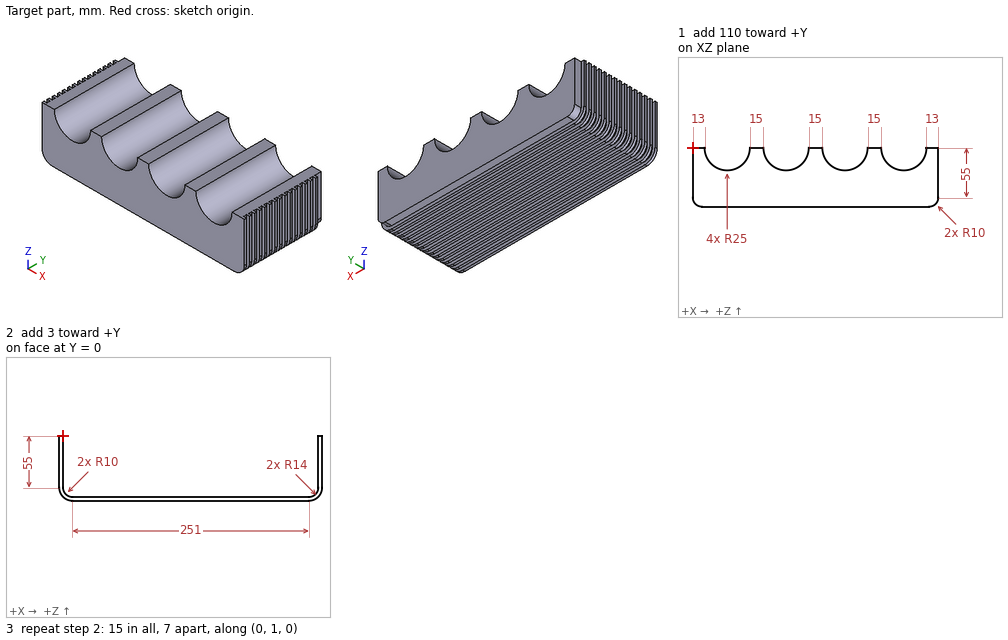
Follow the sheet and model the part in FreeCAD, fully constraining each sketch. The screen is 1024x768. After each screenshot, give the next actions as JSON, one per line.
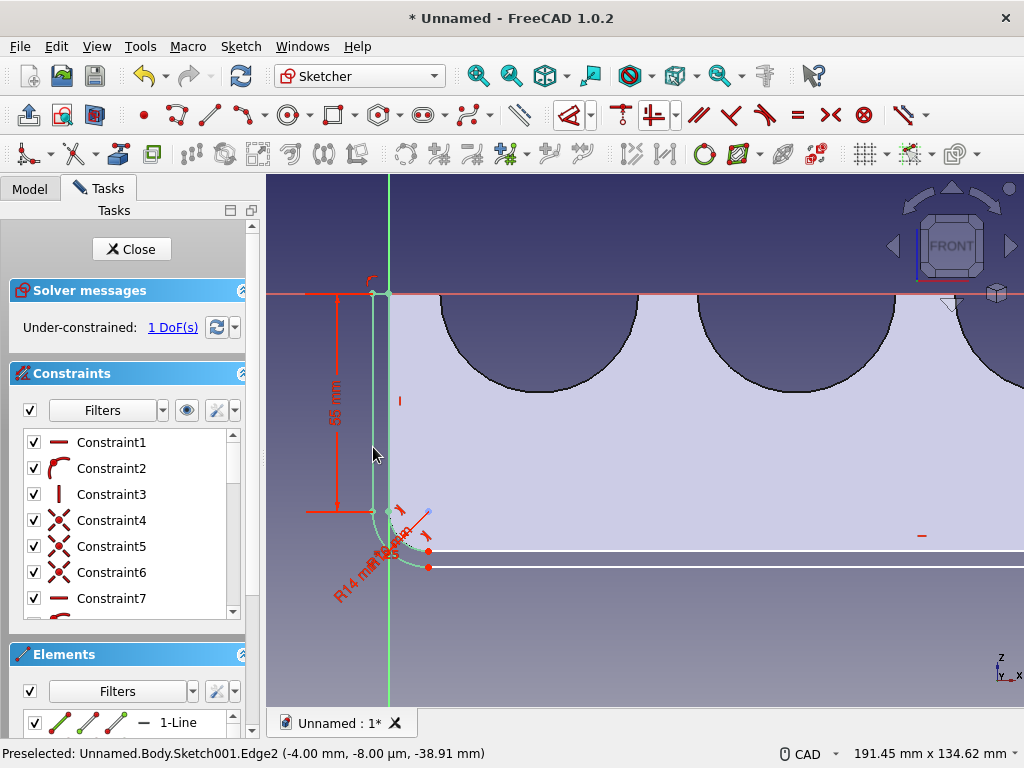
{"action": "left_click", "coordinate": [726, 567]}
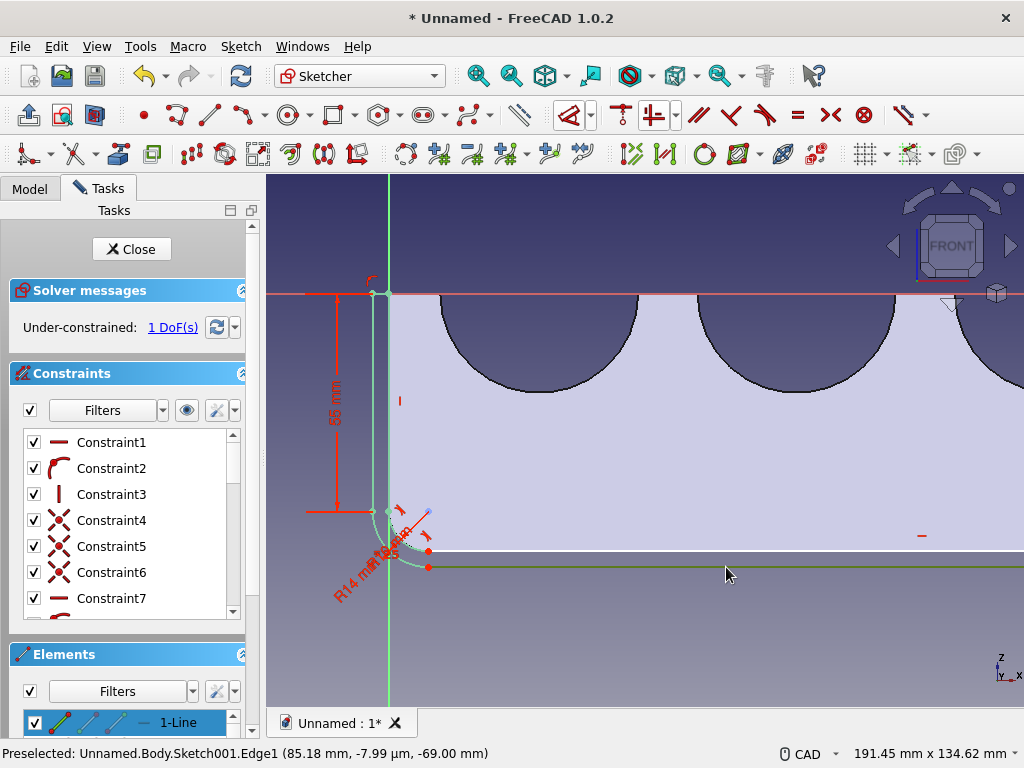
{"action": "key", "text": "l"}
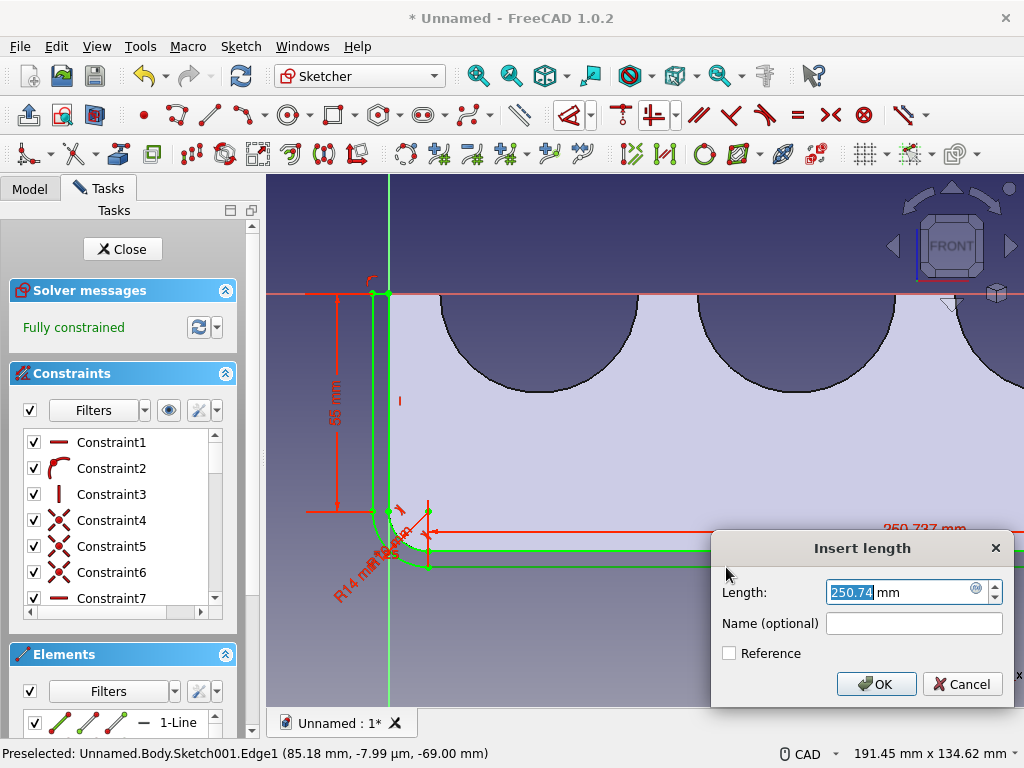
{"action": "type", "text": "251"}
{"action": "key", "text": "Return"}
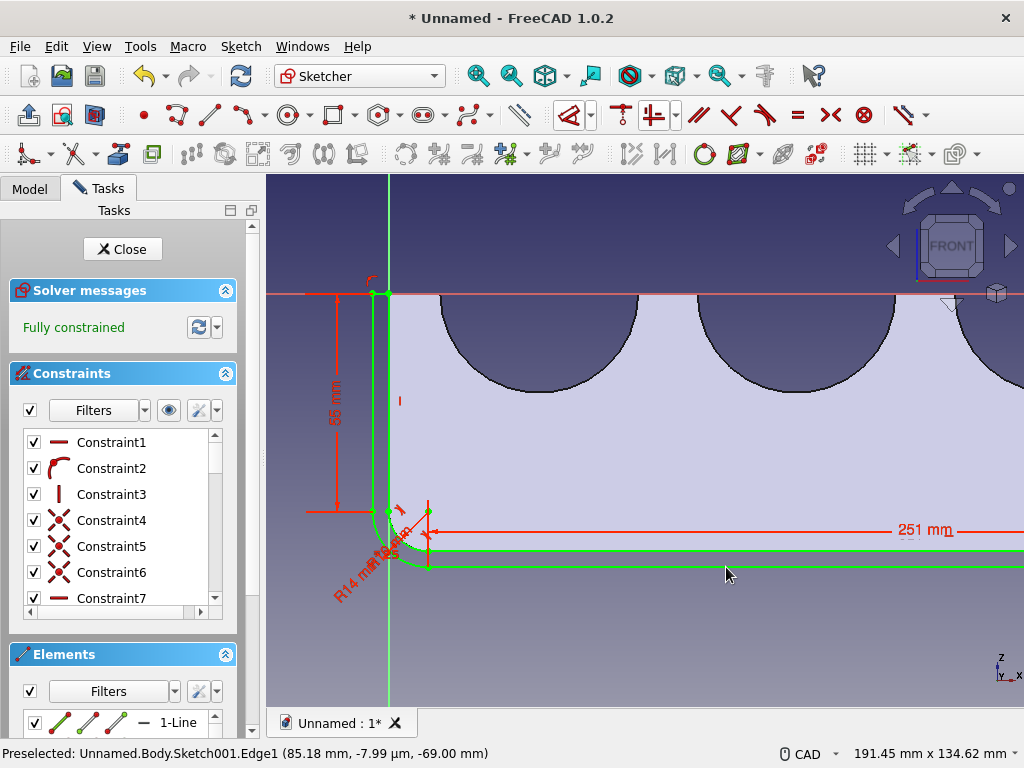
{"action": "left_click", "coordinate": [123, 249]}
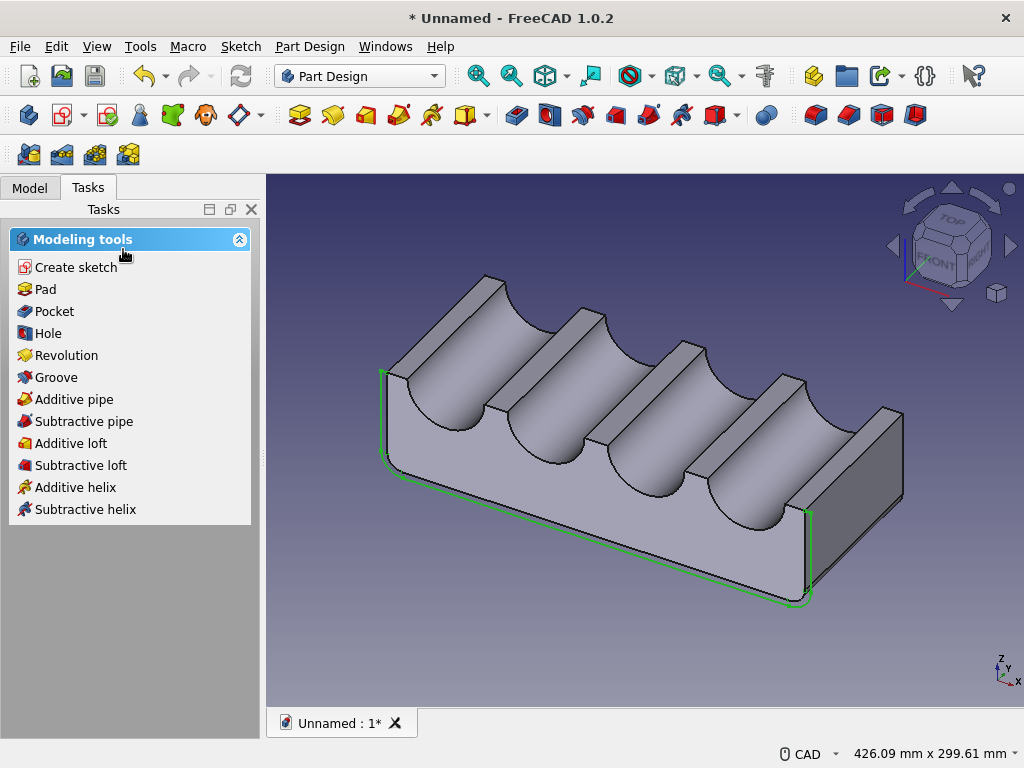
{"action": "left_click", "coordinate": [300, 116]}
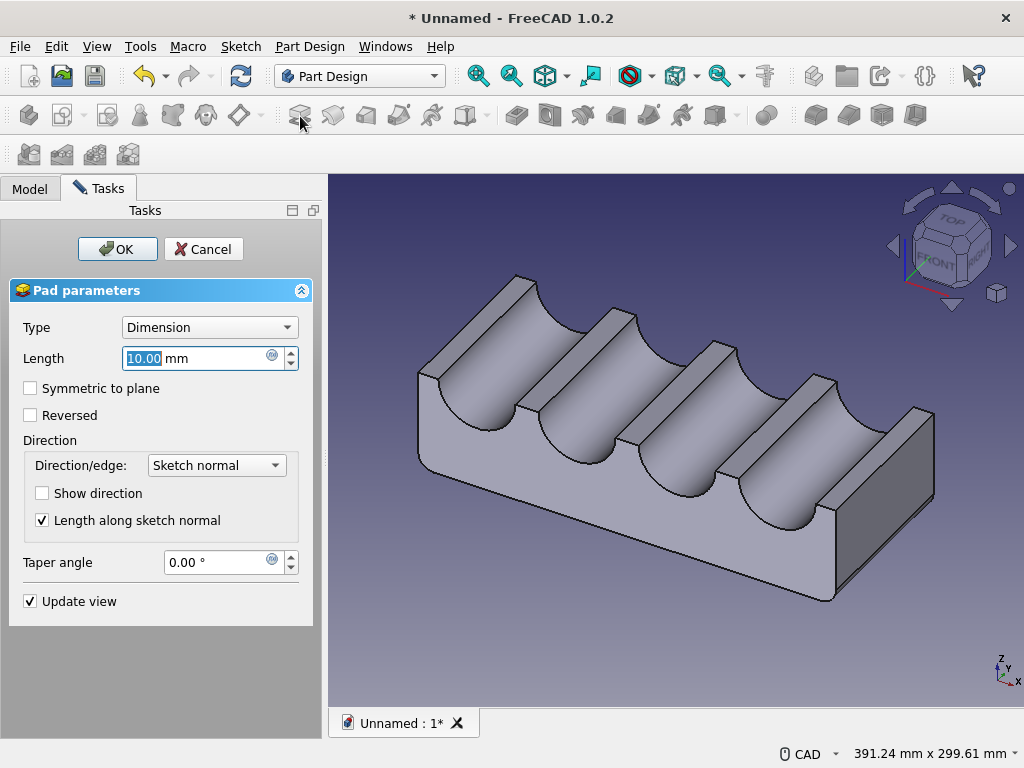
{"action": "type", "text": "3"}
{"action": "key", "text": "Tab"}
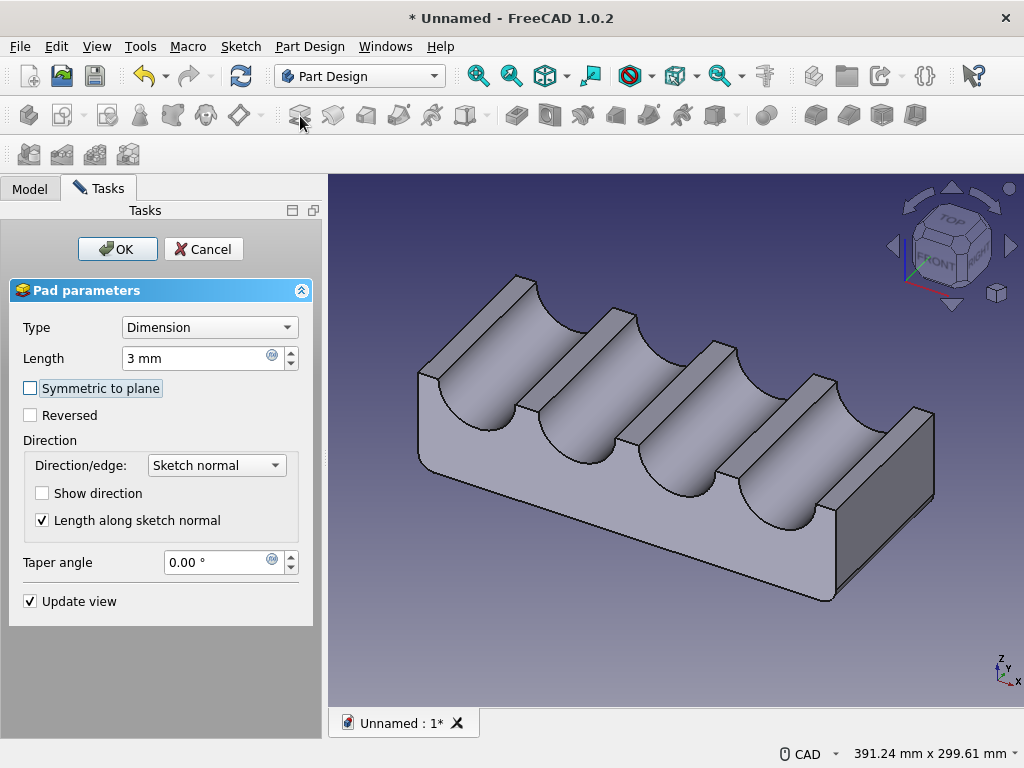
{"action": "left_click", "coordinate": [31, 415]}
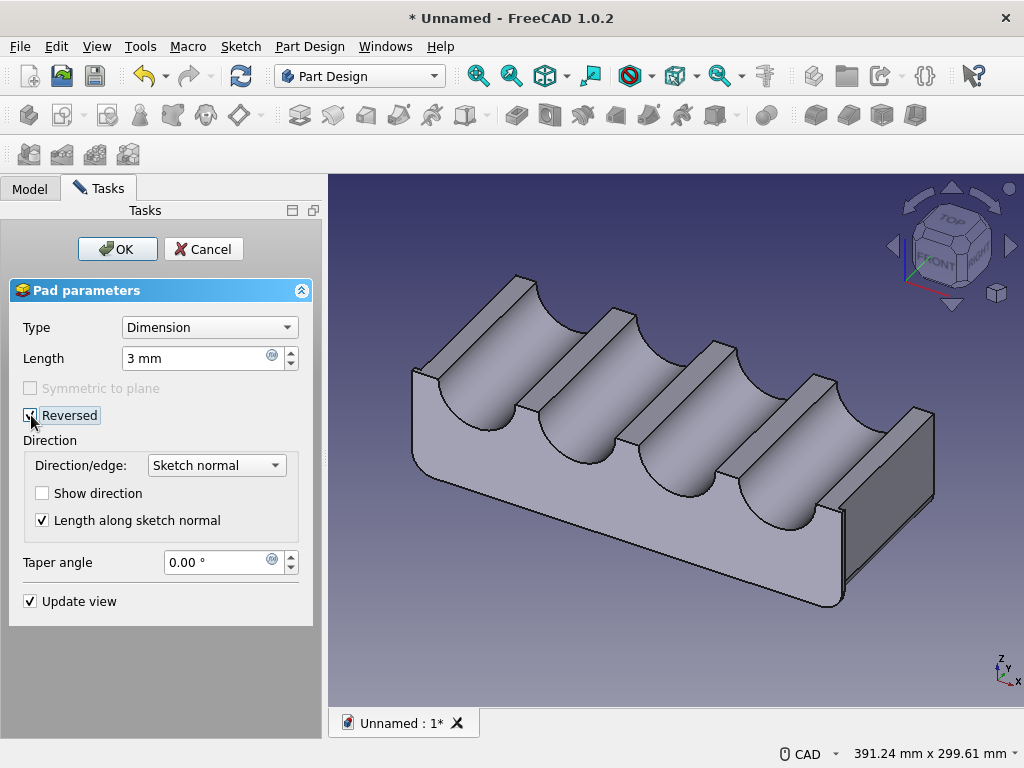
{"action": "left_click", "coordinate": [118, 249]}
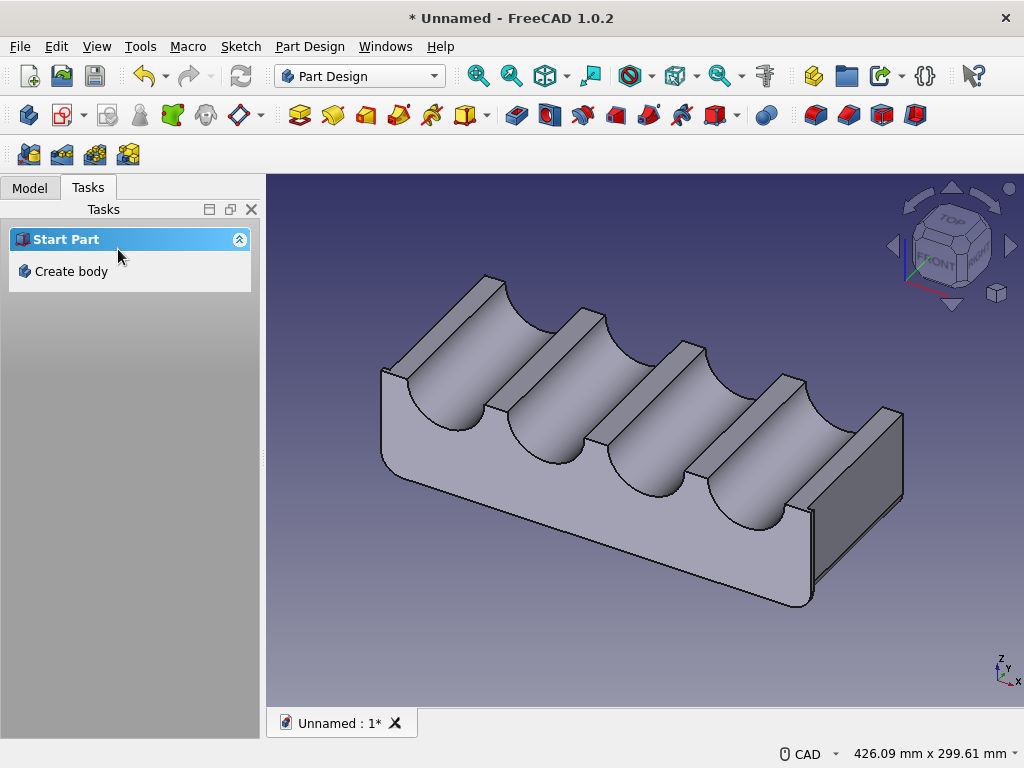
{"action": "left_click", "coordinate": [30, 188]}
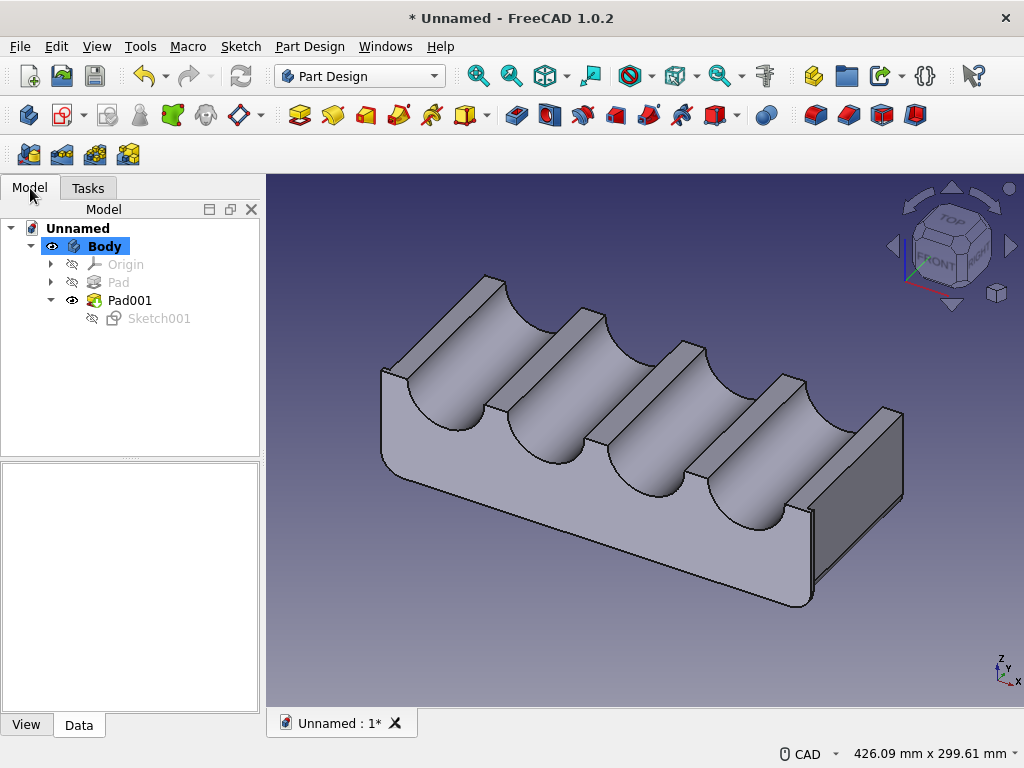
{"action": "left_click", "coordinate": [117, 300]}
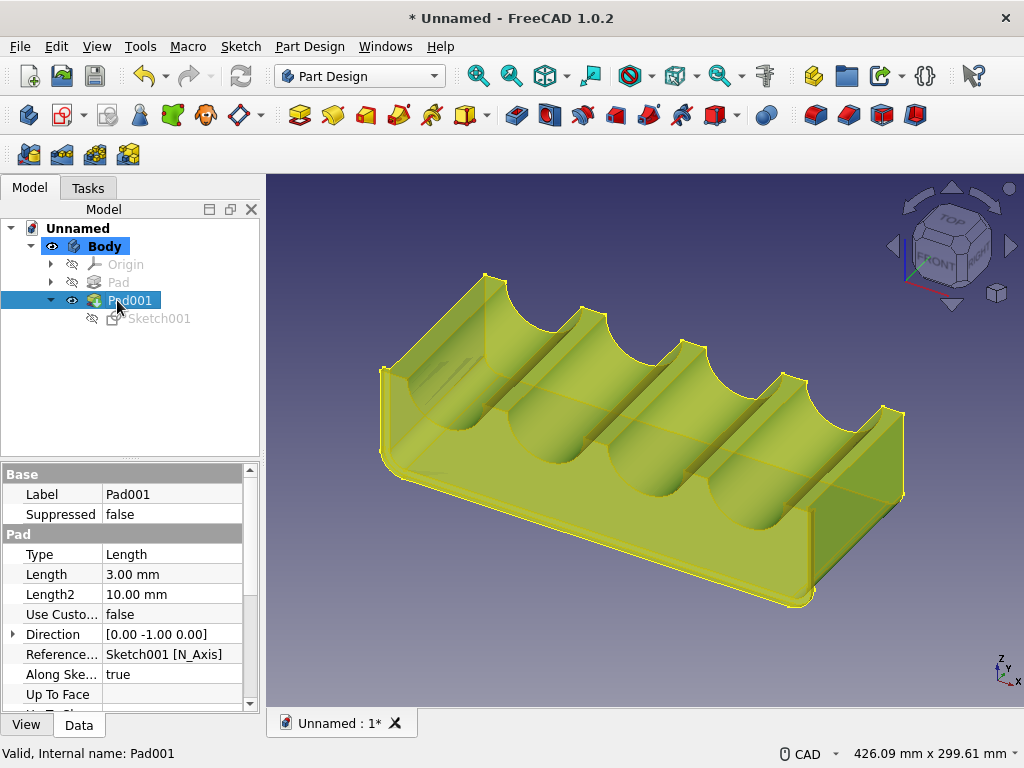
{"action": "left_click", "coordinate": [62, 154]}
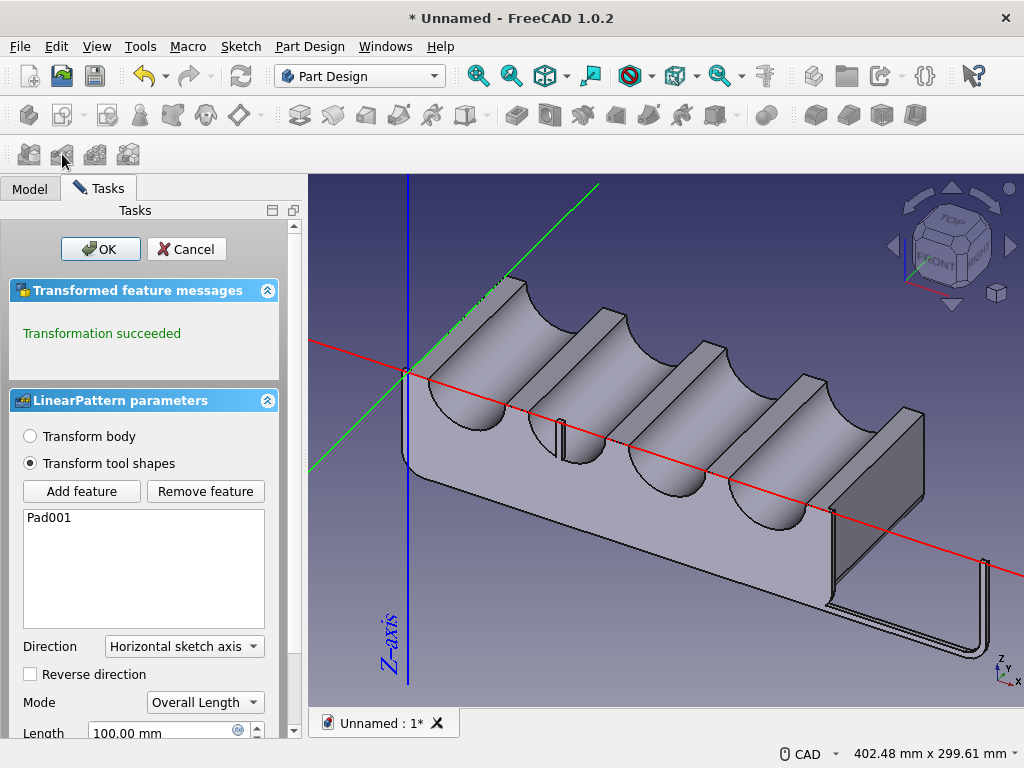
{"action": "left_click", "coordinate": [185, 646]}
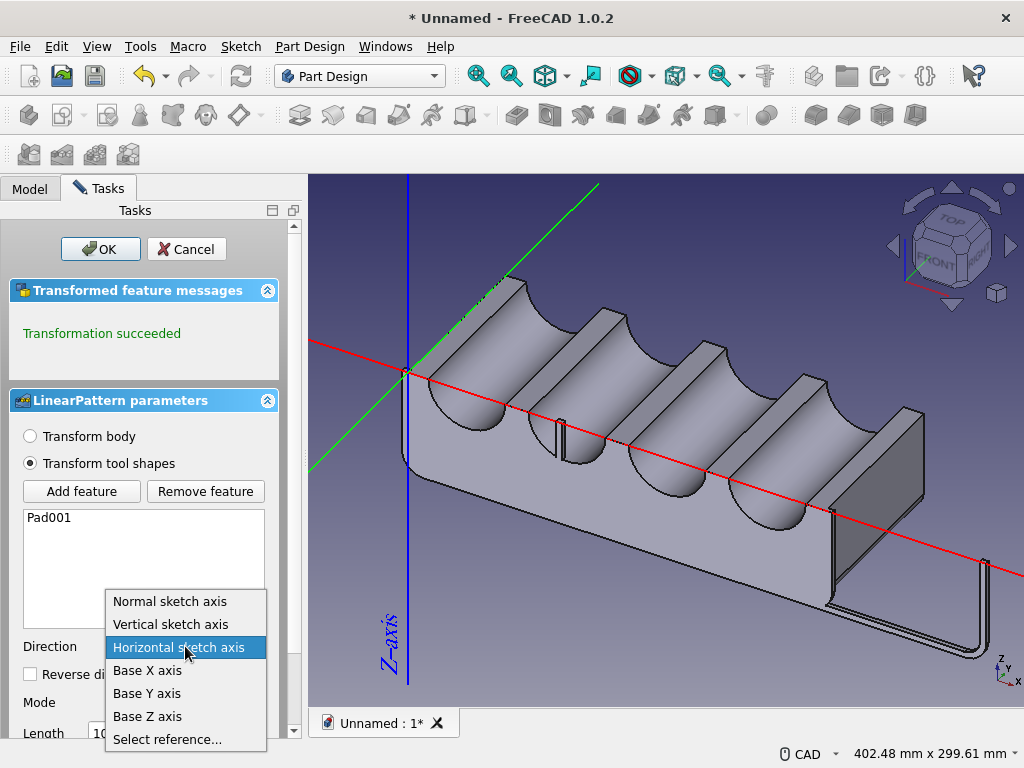
{"action": "left_click", "coordinate": [184, 694]}